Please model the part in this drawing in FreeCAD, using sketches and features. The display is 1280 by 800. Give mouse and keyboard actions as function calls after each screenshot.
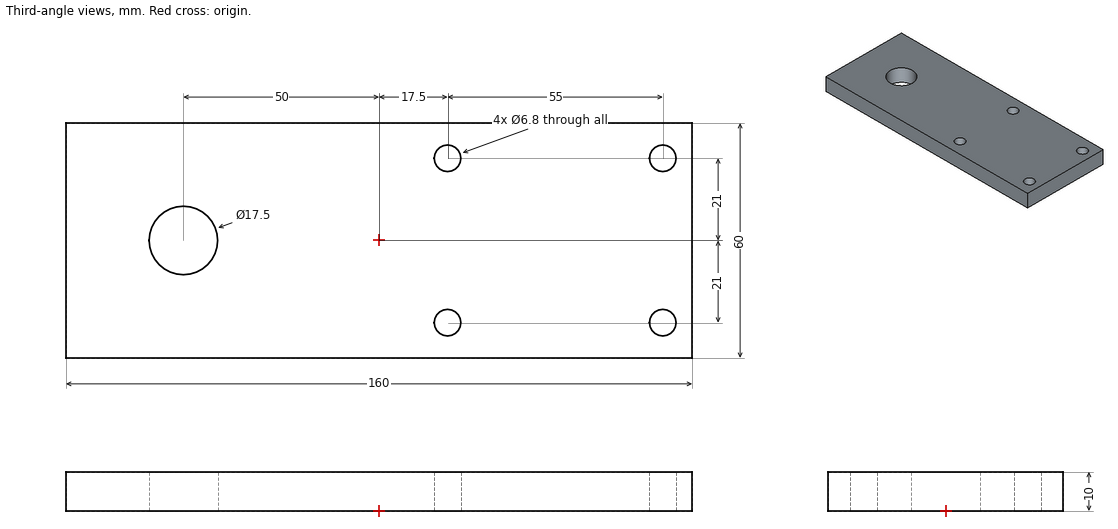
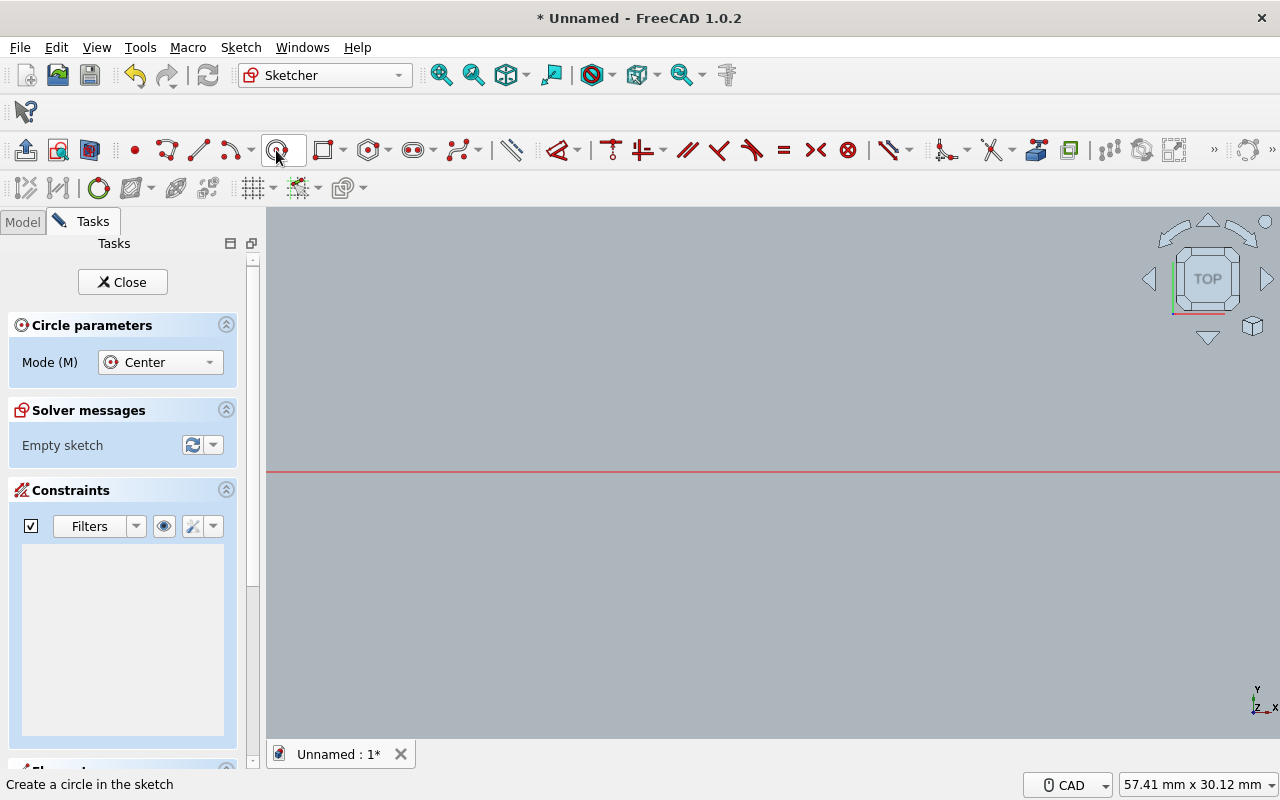
click(705, 472)
click(815, 363)
key(Escape)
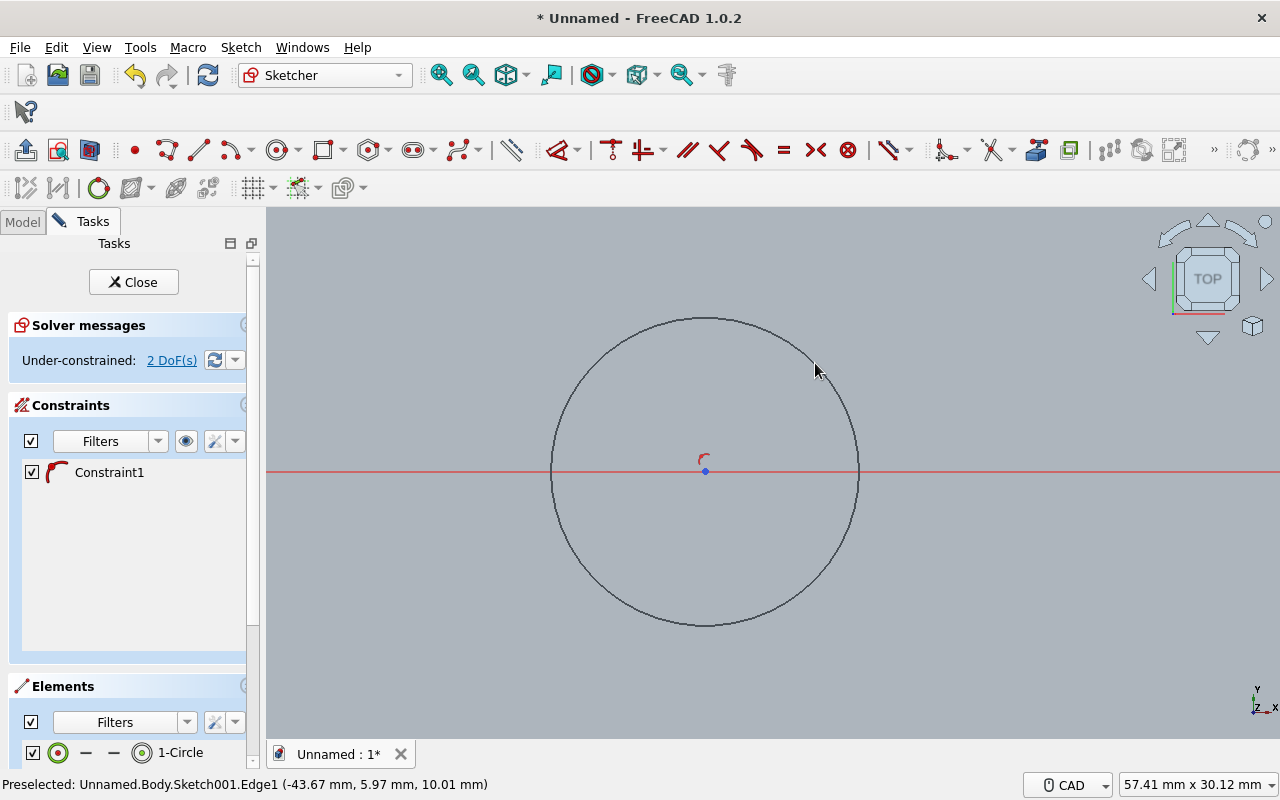
click(558, 150)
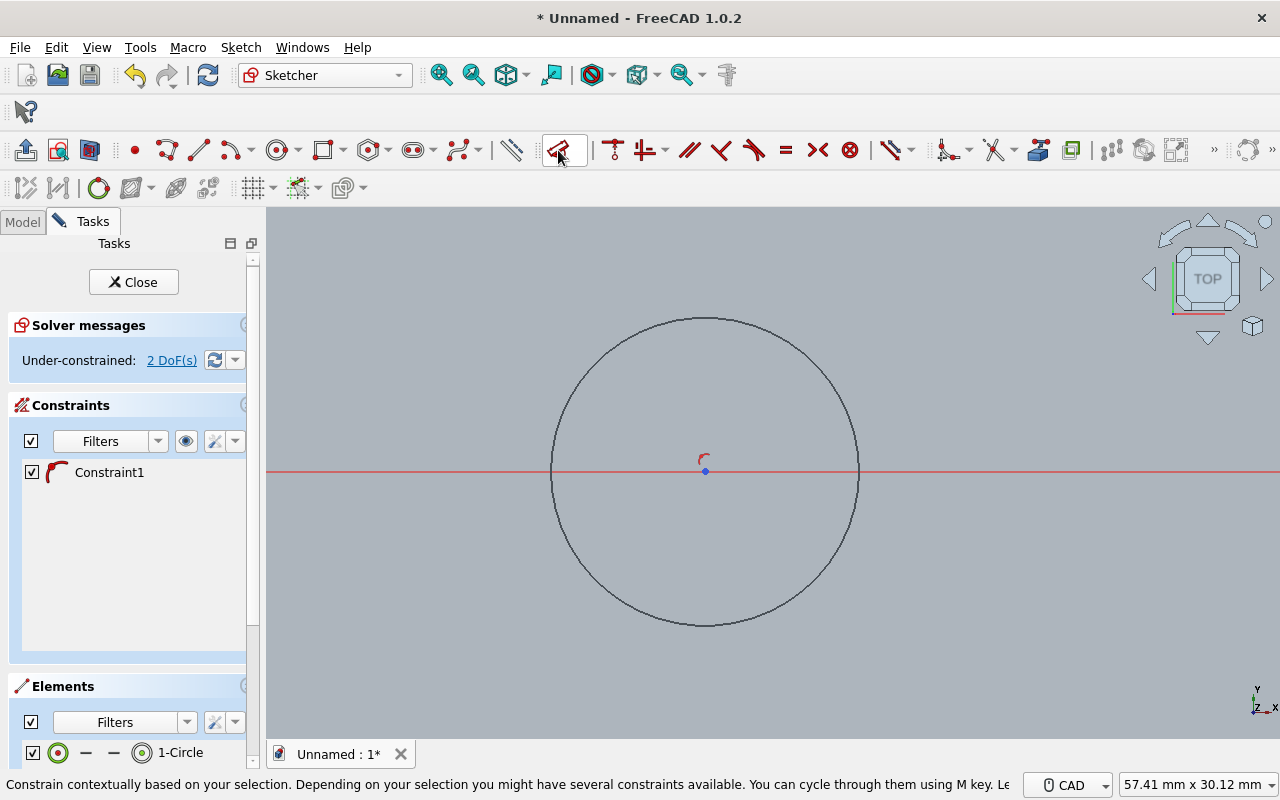
click(814, 363)
click(837, 340)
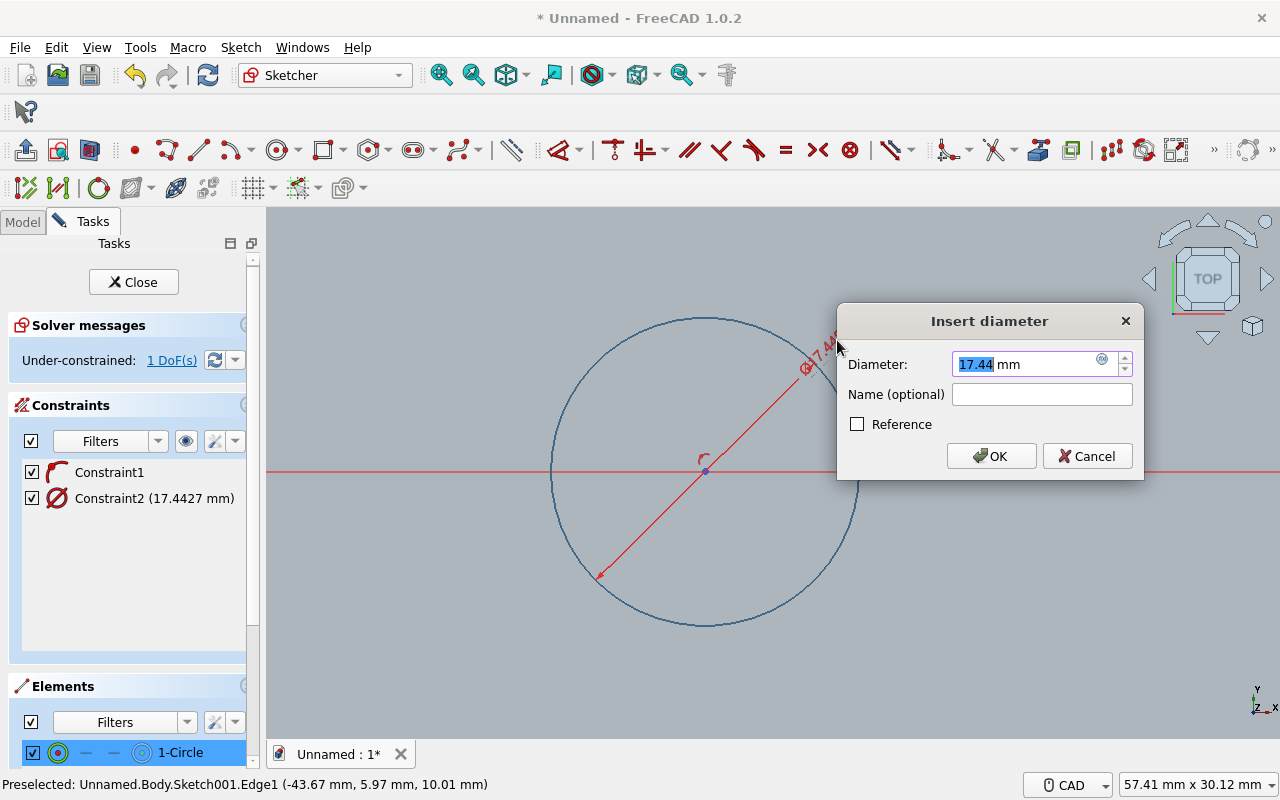
text(17.5)
key(Return)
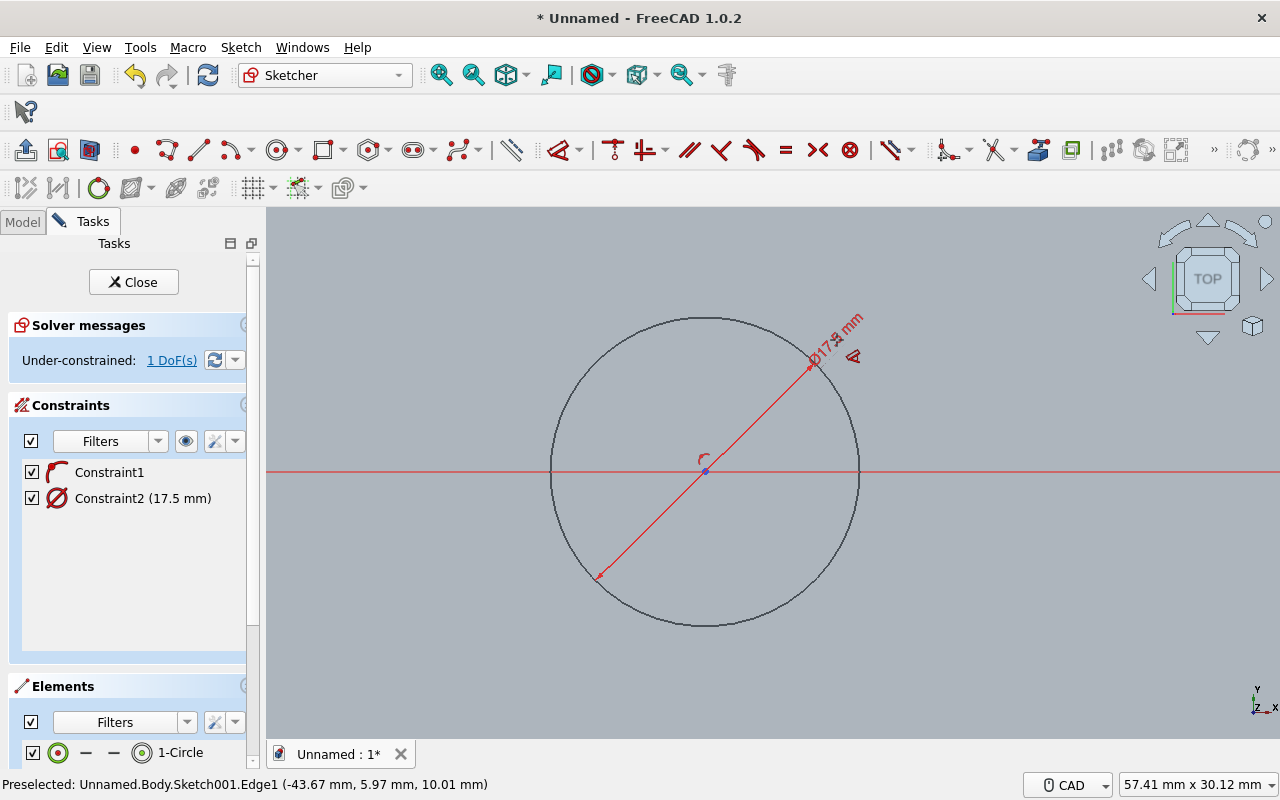
click(705, 472)
click(910, 506)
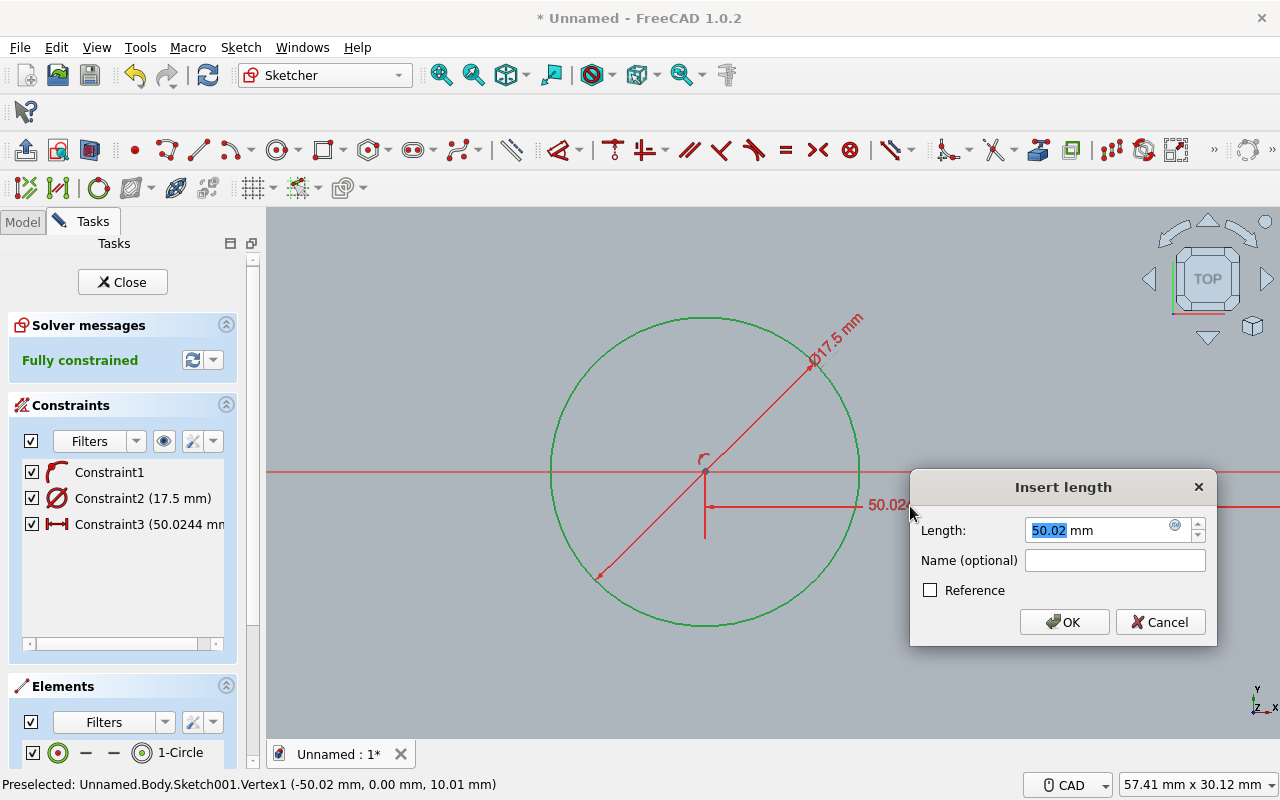
text(50)
key(Return)
key(Escape)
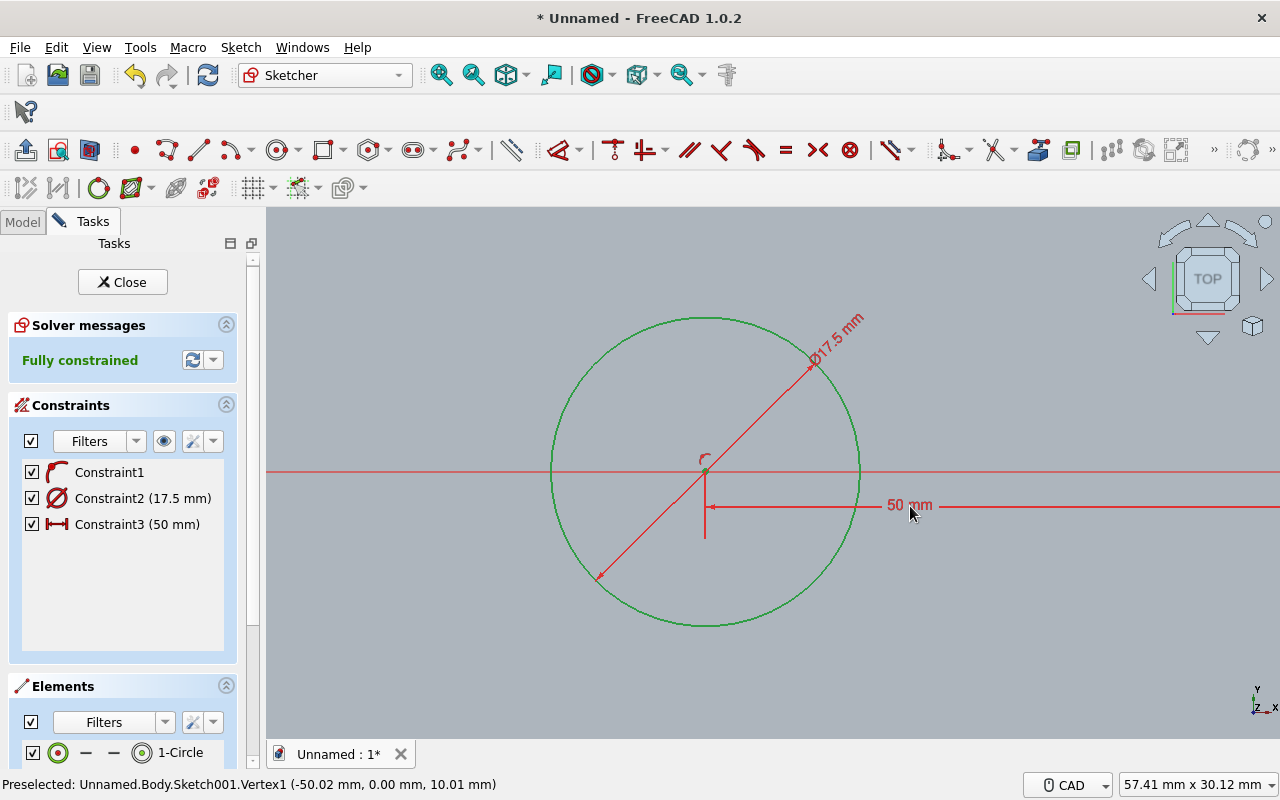
click(123, 282)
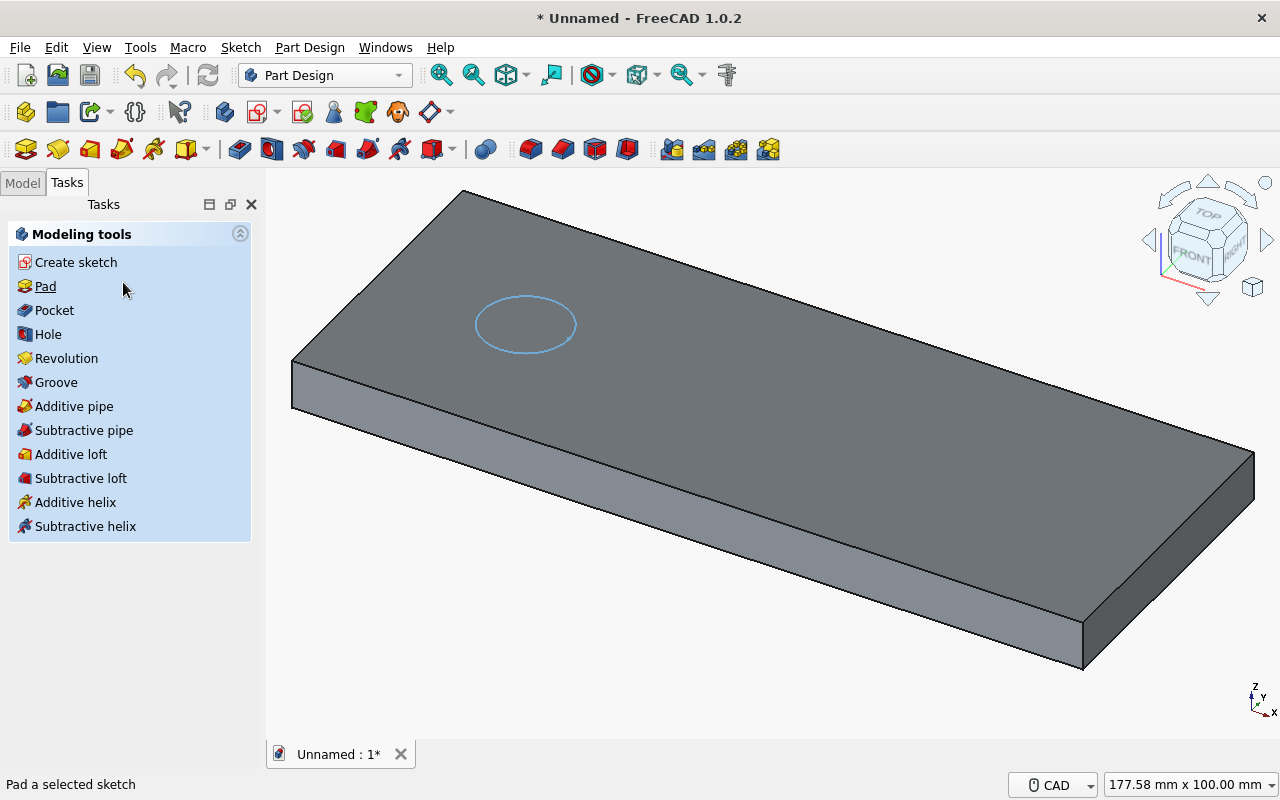
click(240, 150)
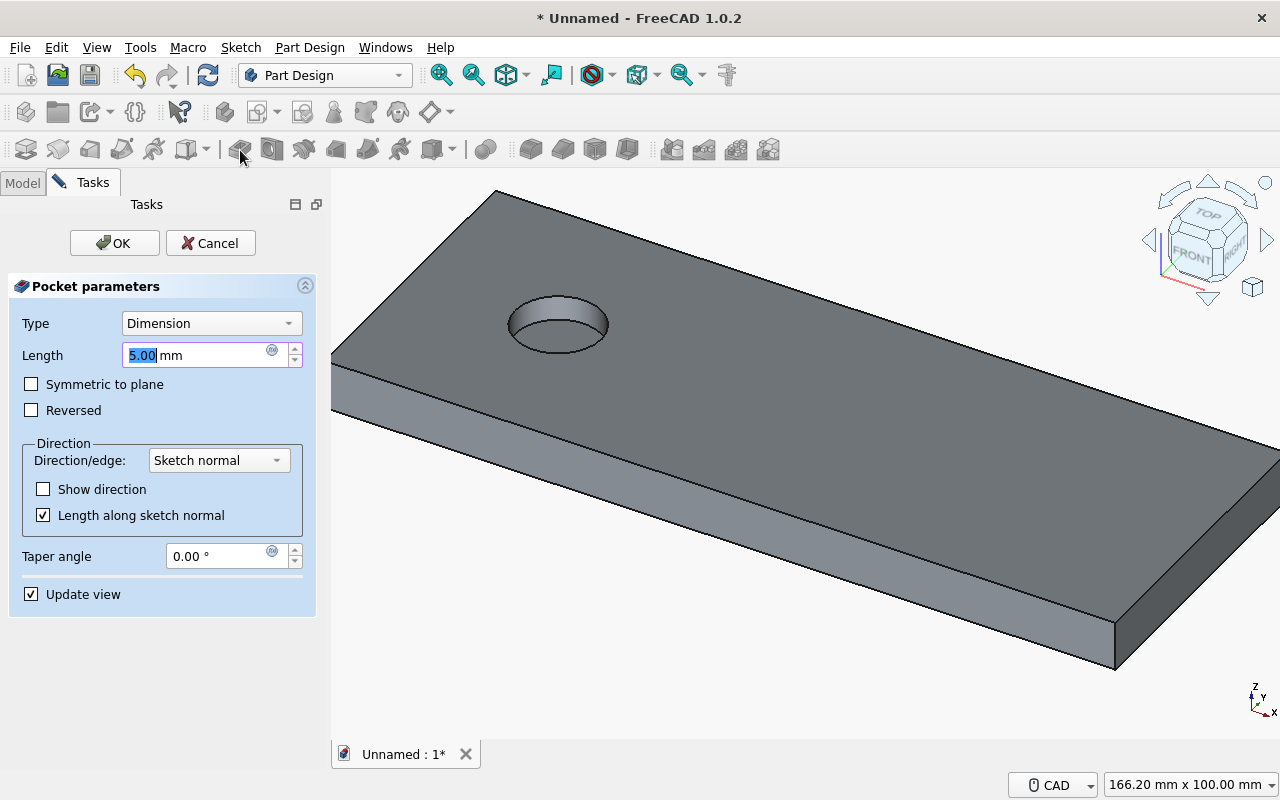
click(212, 324)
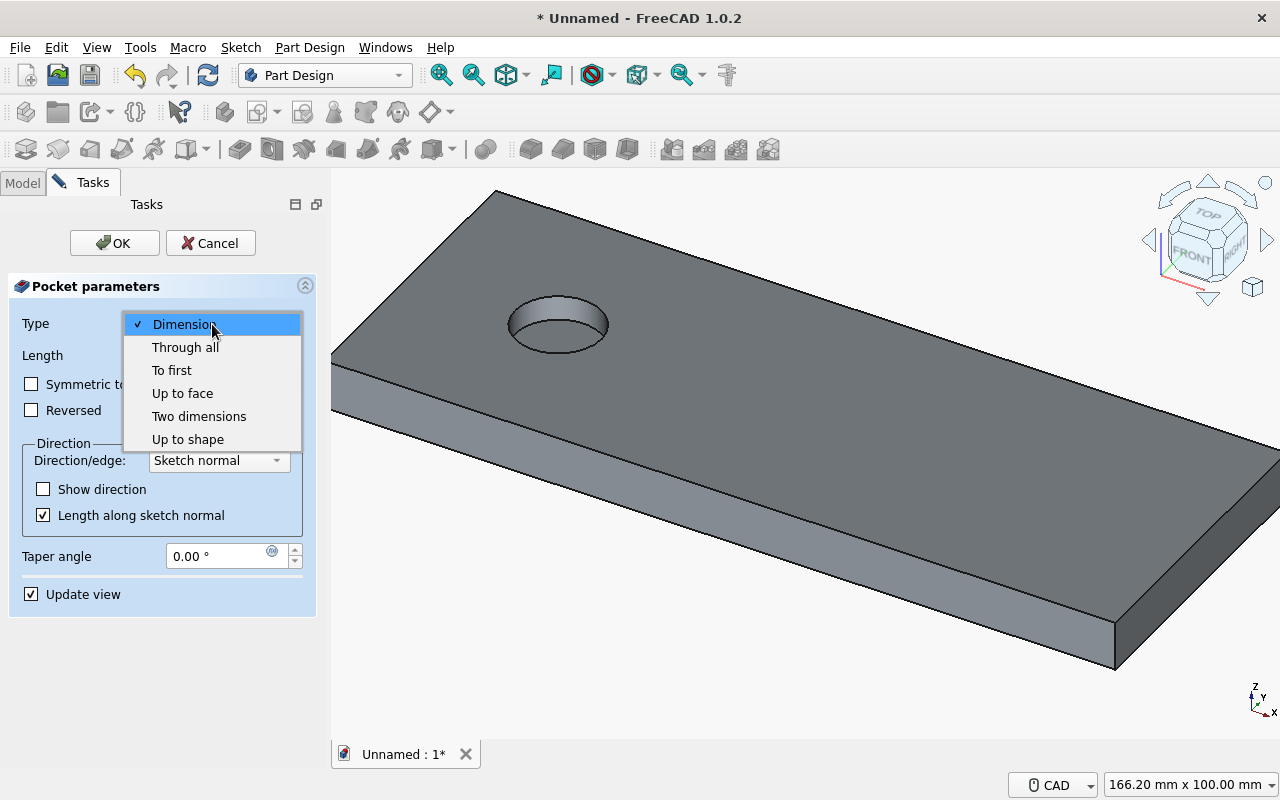
click(212, 348)